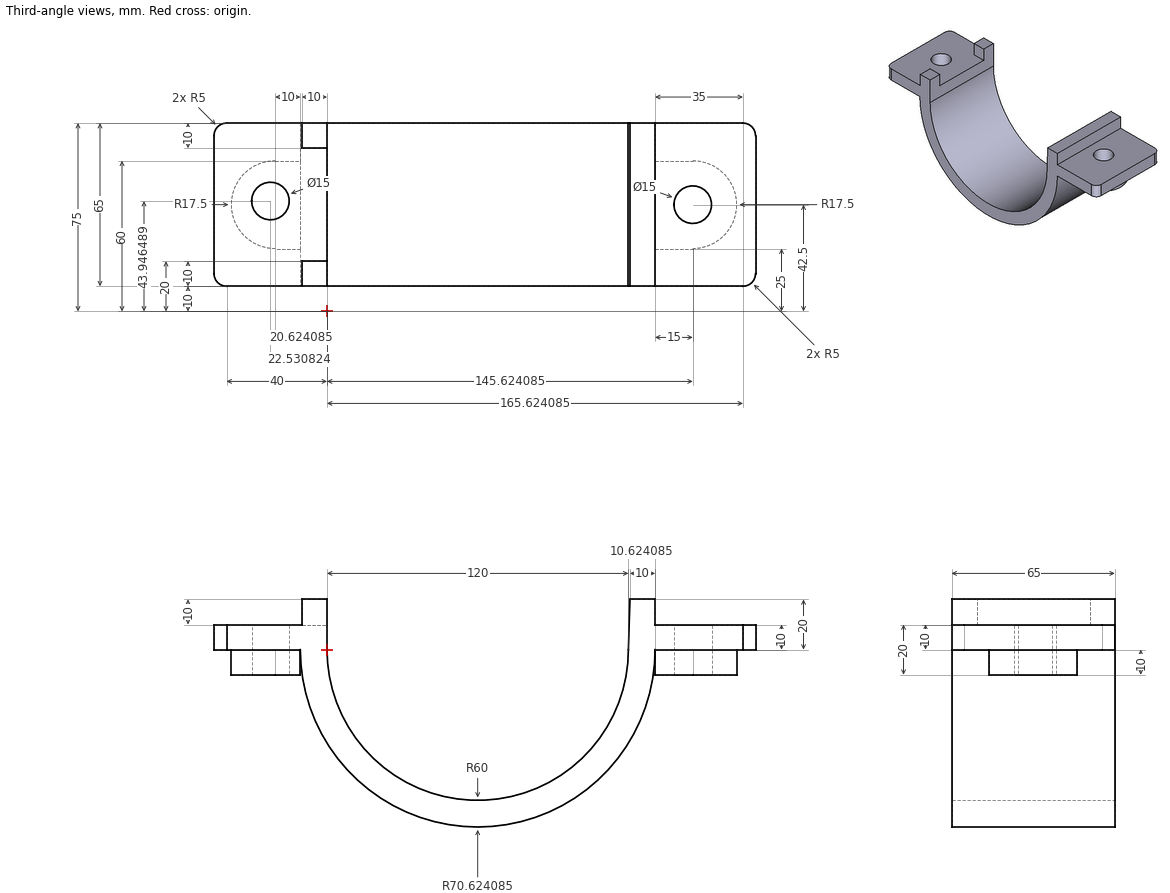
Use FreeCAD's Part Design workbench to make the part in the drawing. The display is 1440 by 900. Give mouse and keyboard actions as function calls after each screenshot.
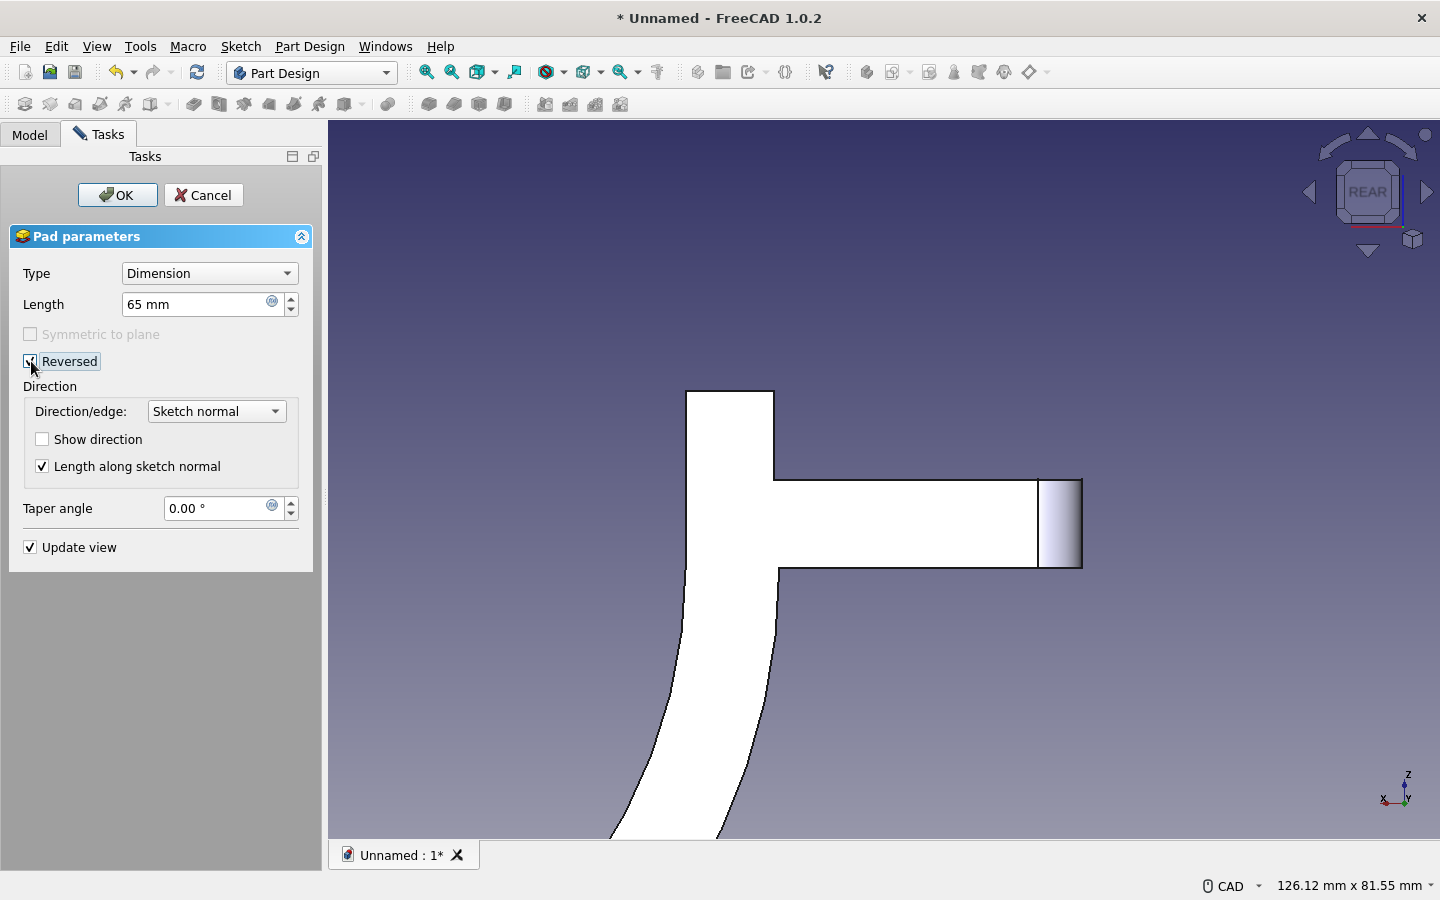
click(118, 195)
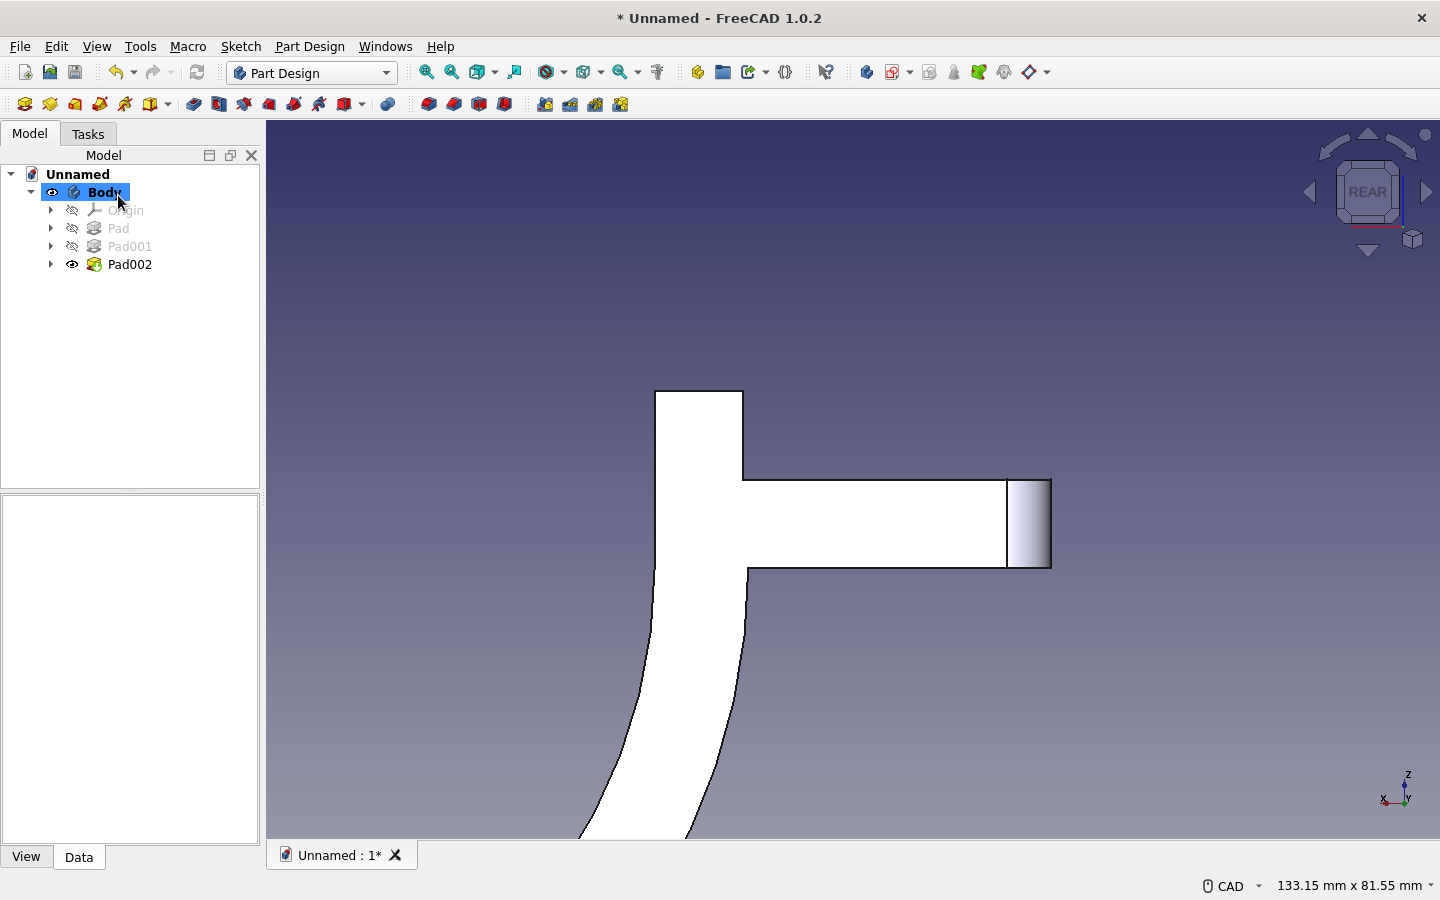
click(427, 72)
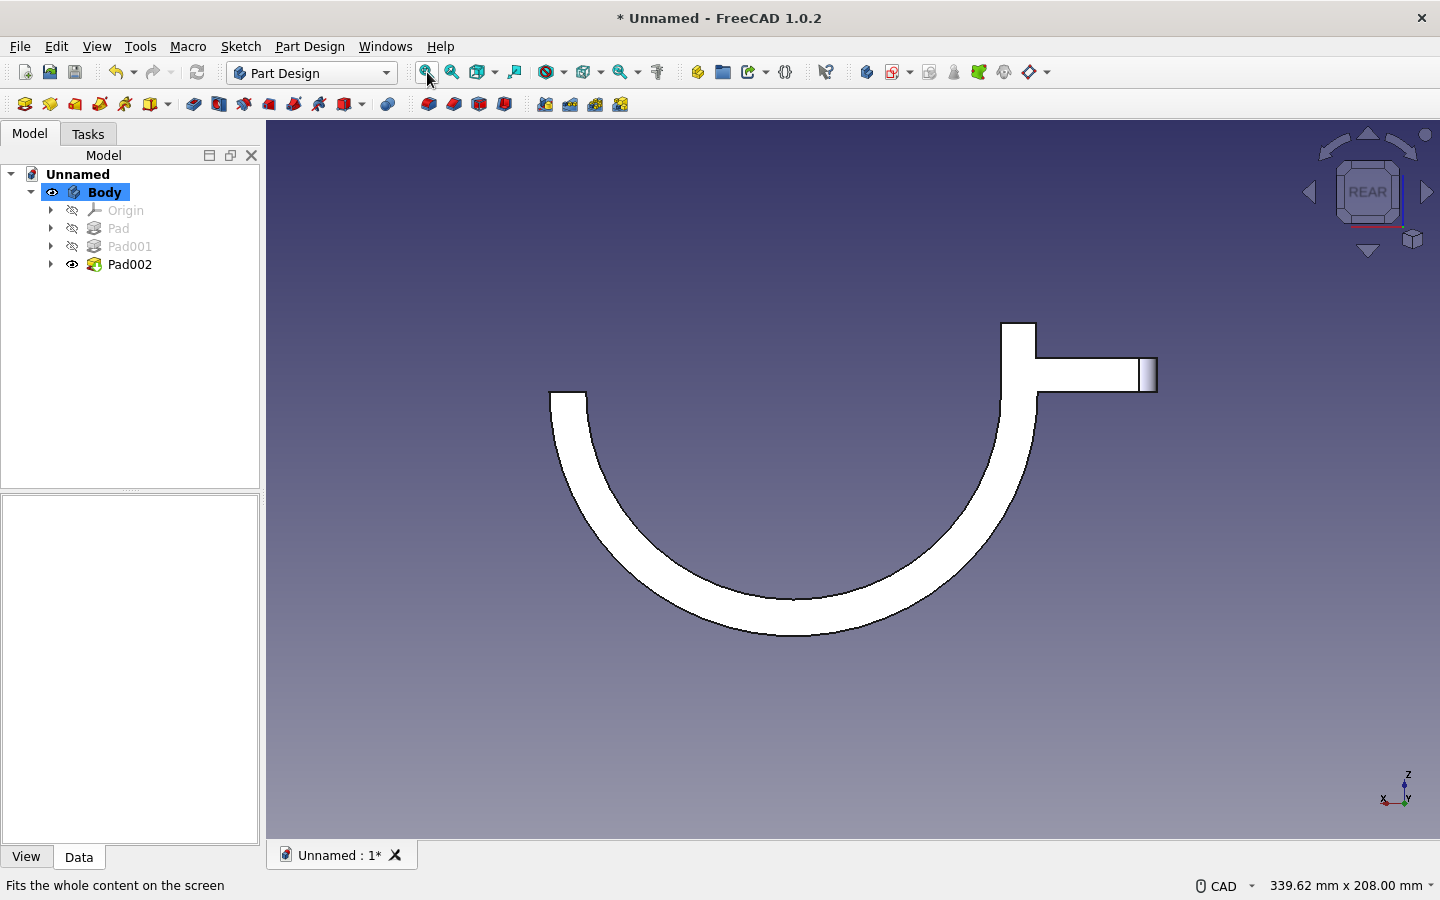
click(867, 72)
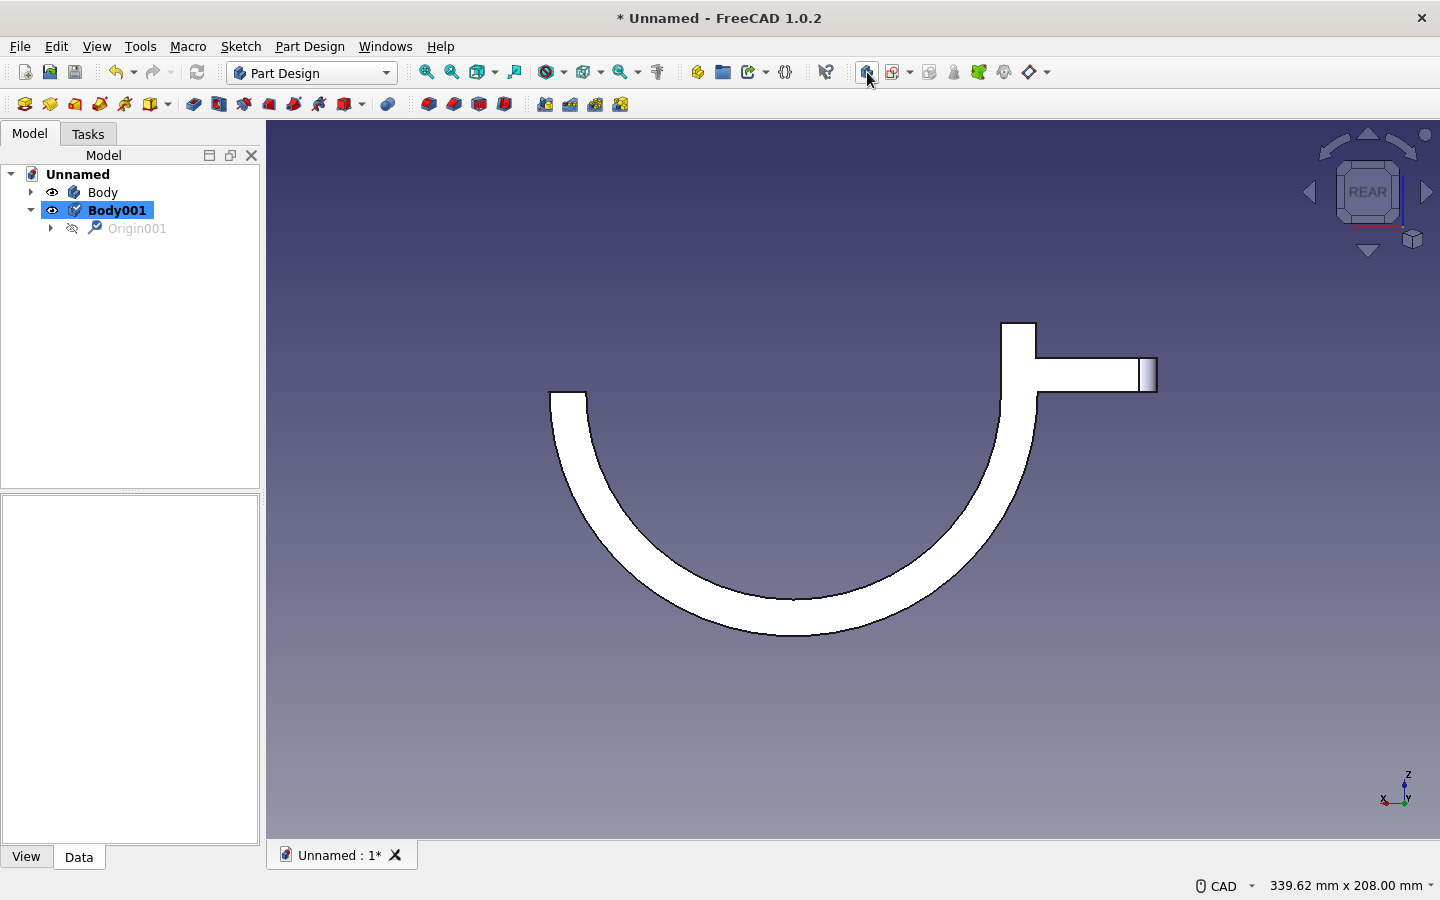
click(306, 799)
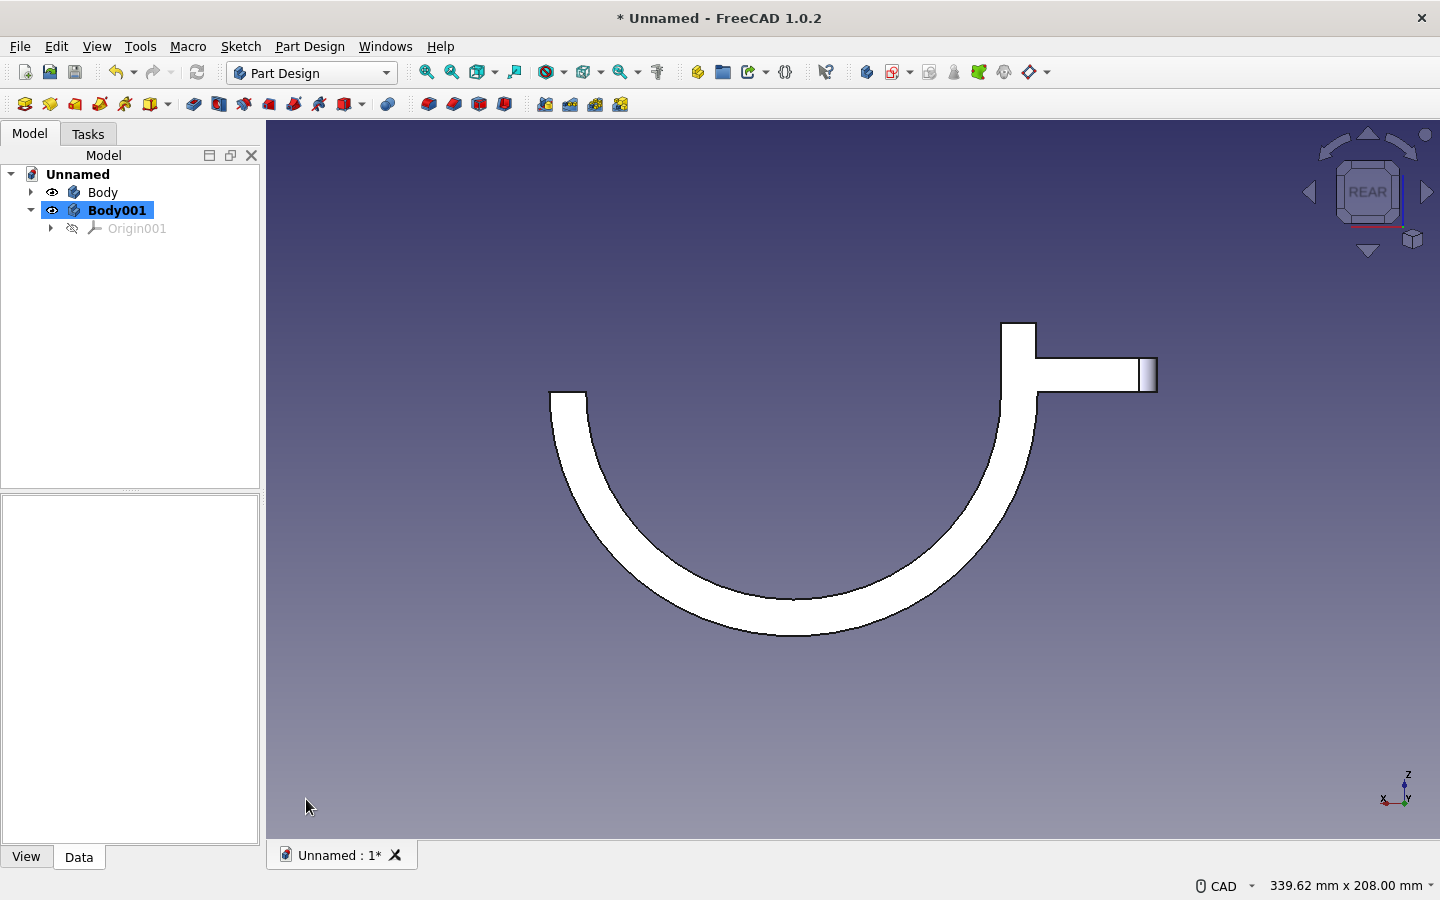
click(892, 72)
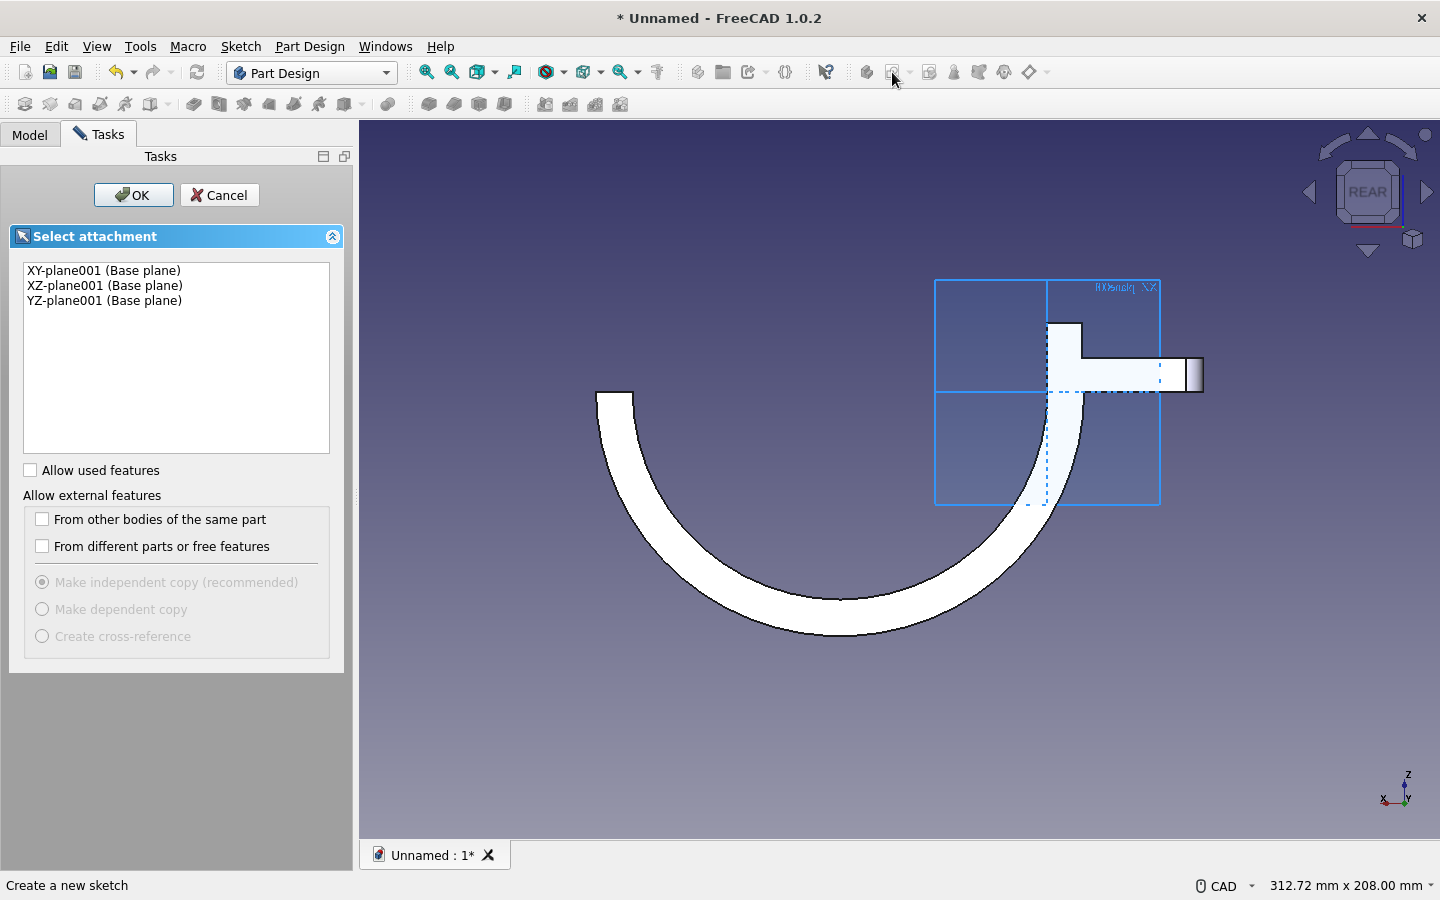
click(84, 270)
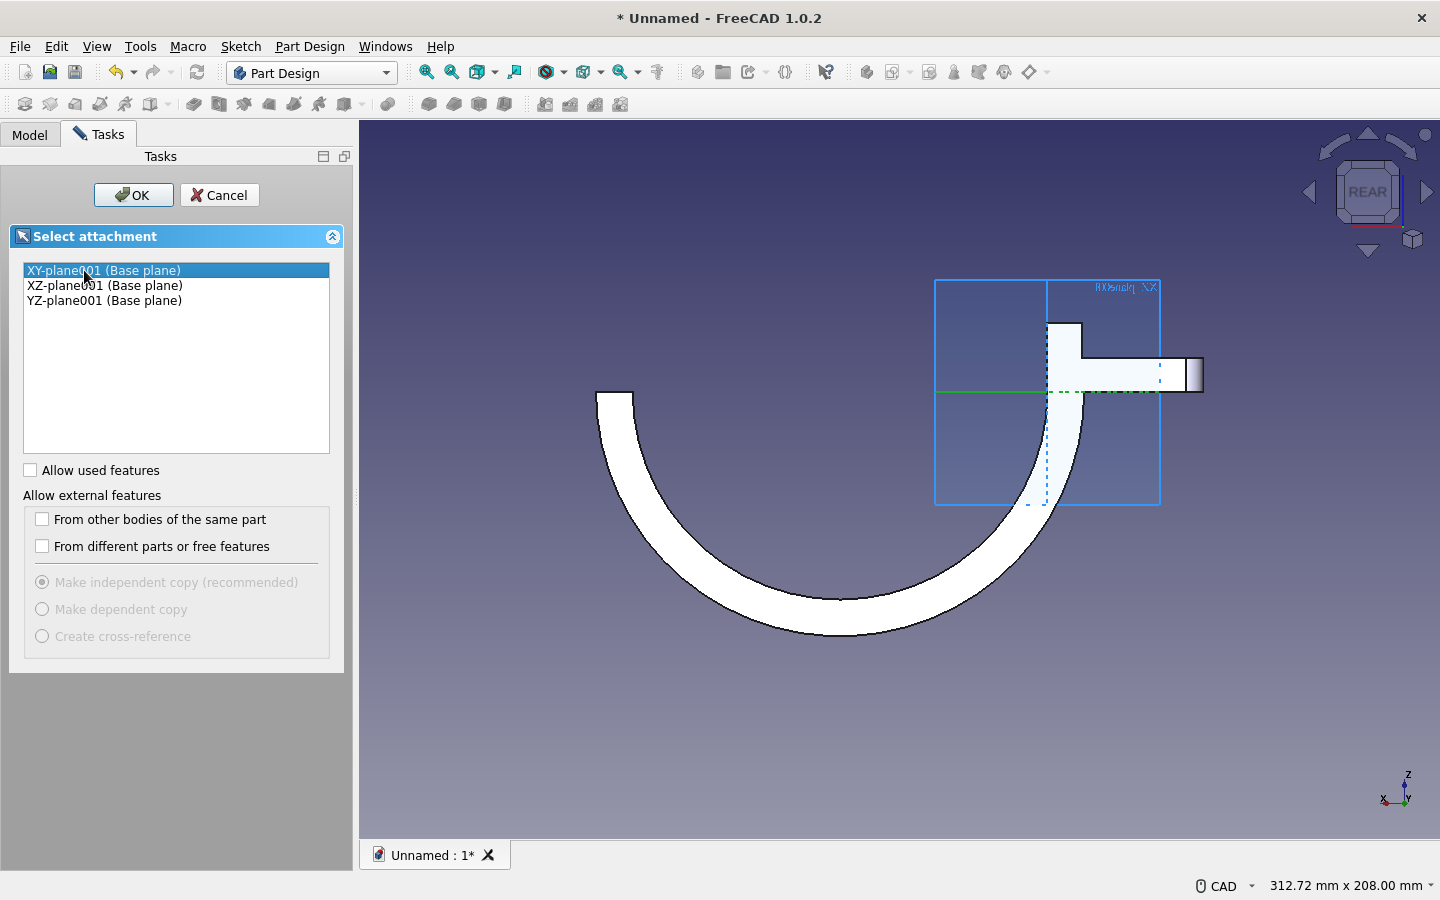
click(134, 195)